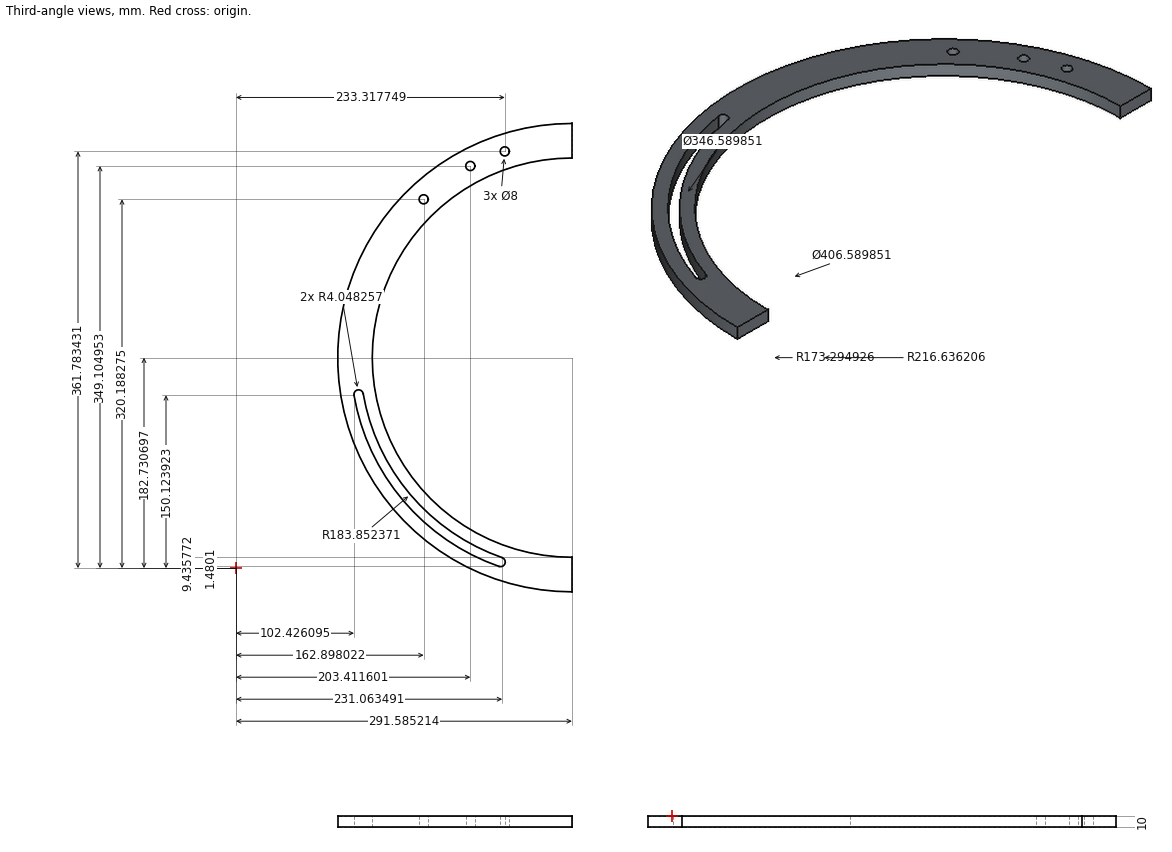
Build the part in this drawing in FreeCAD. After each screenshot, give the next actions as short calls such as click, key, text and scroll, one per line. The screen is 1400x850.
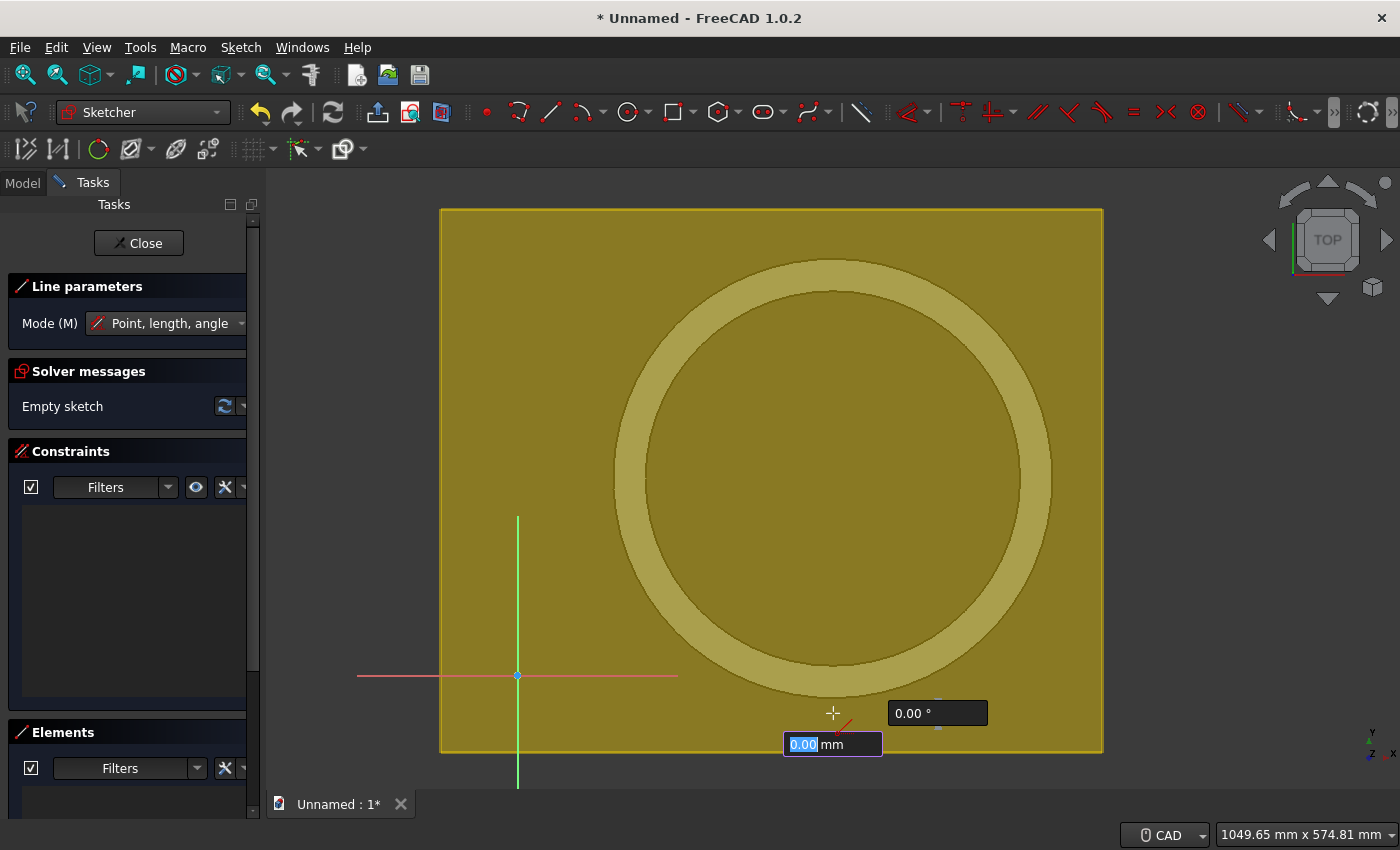
scroll(833, 666, up, 3)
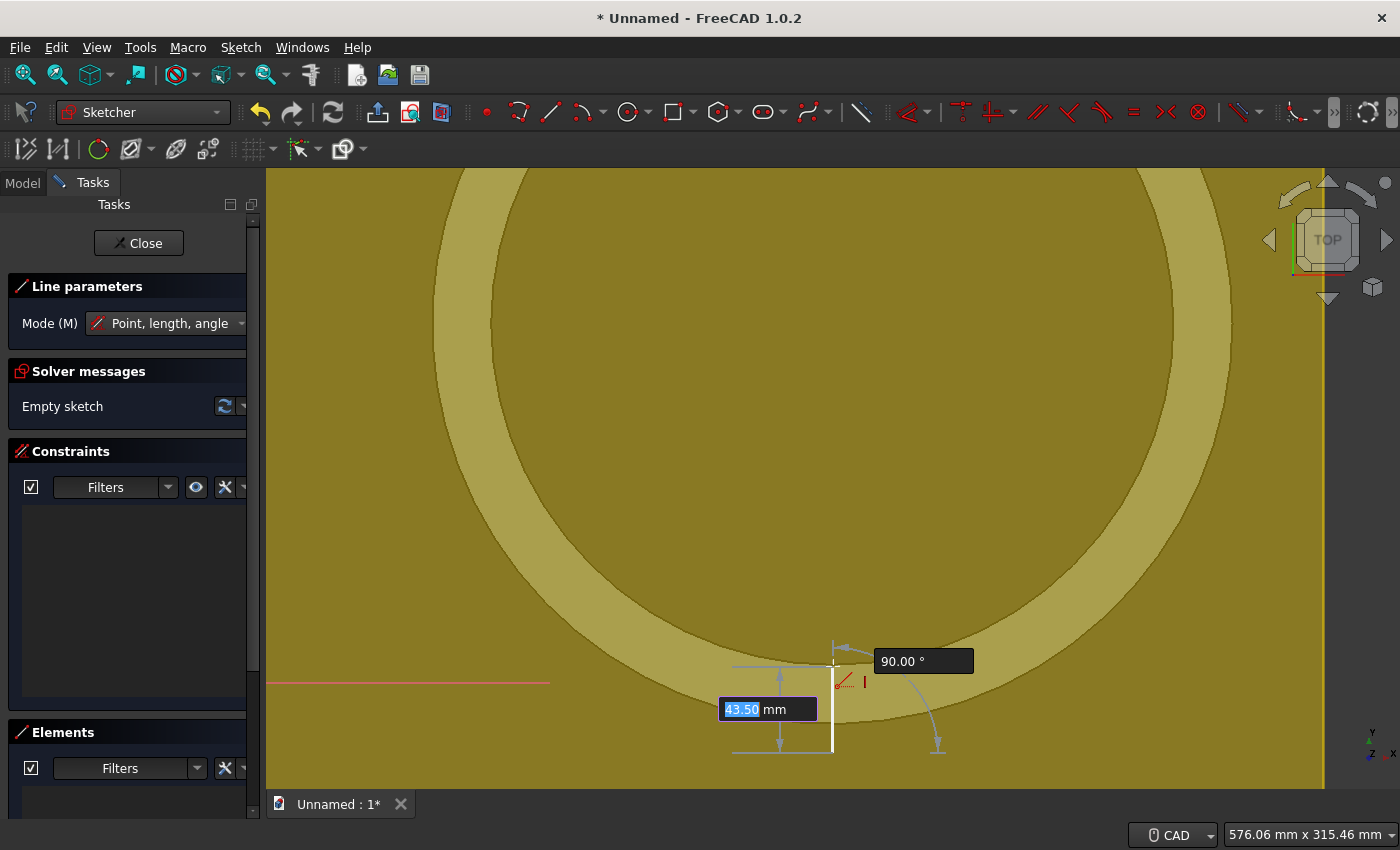
click(833, 665)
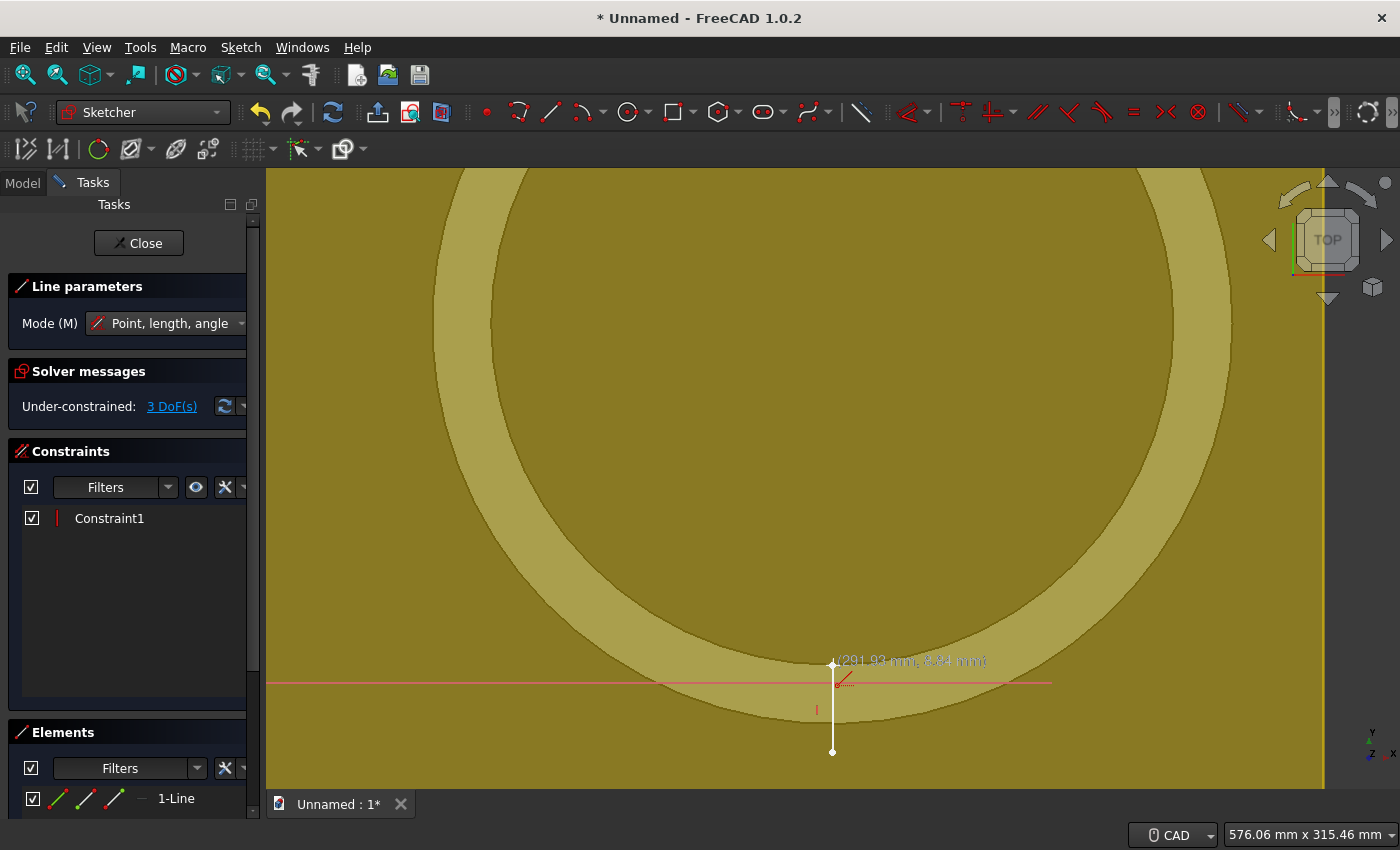
scroll(769, 605, down, 4)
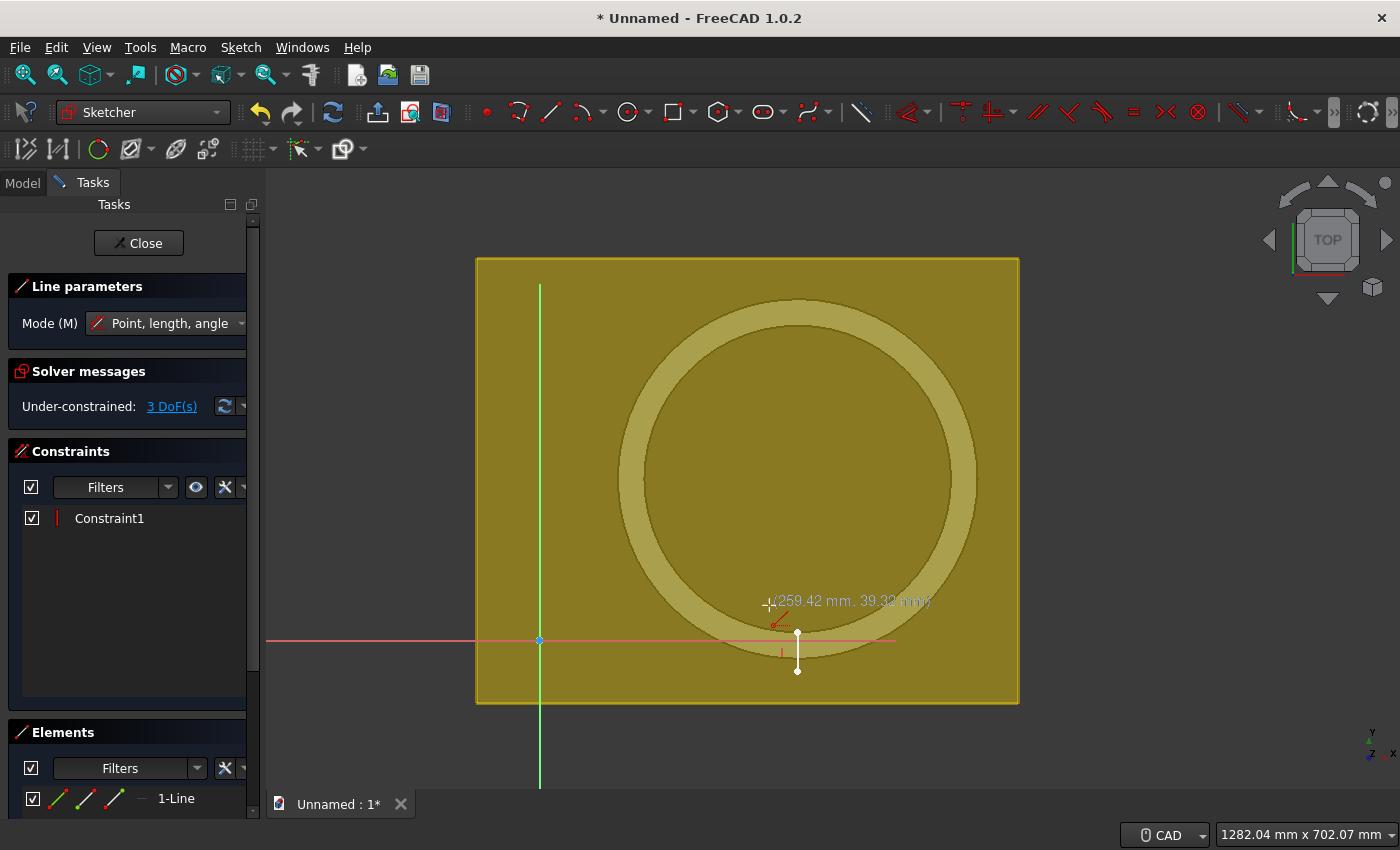
click(798, 326)
click(798, 287)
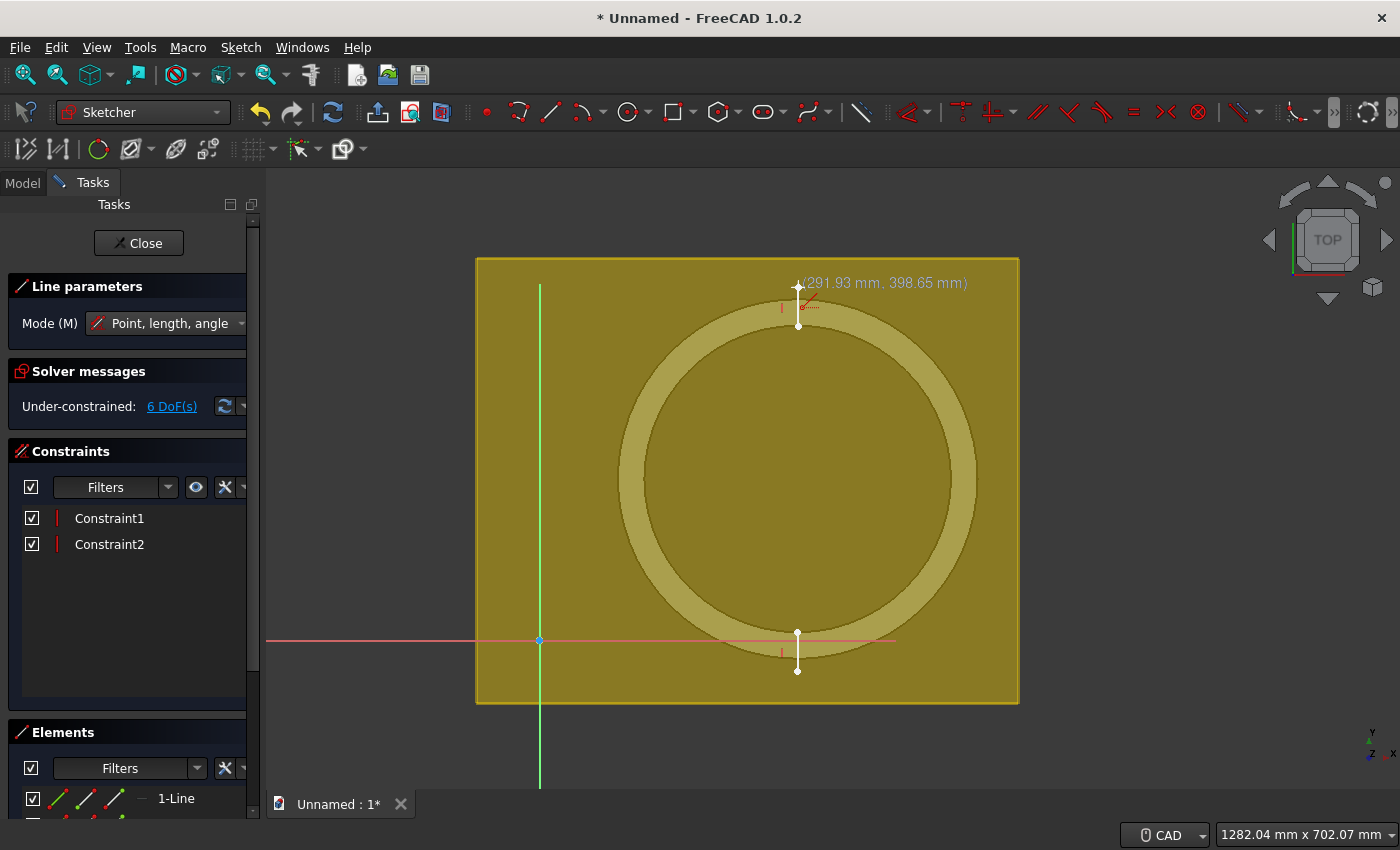
key(g)
key(3)
key(a)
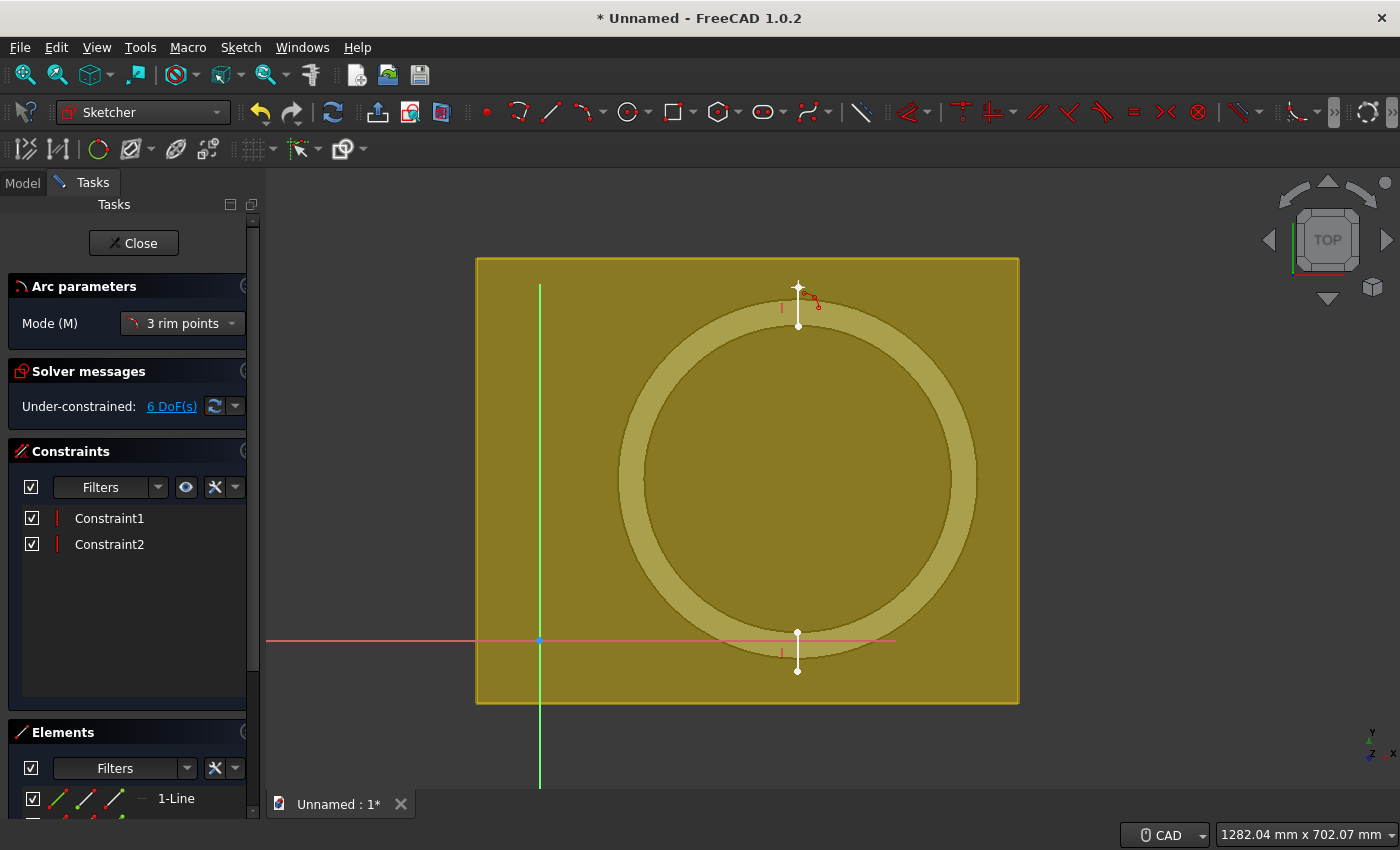
scroll(798, 632, up, 4)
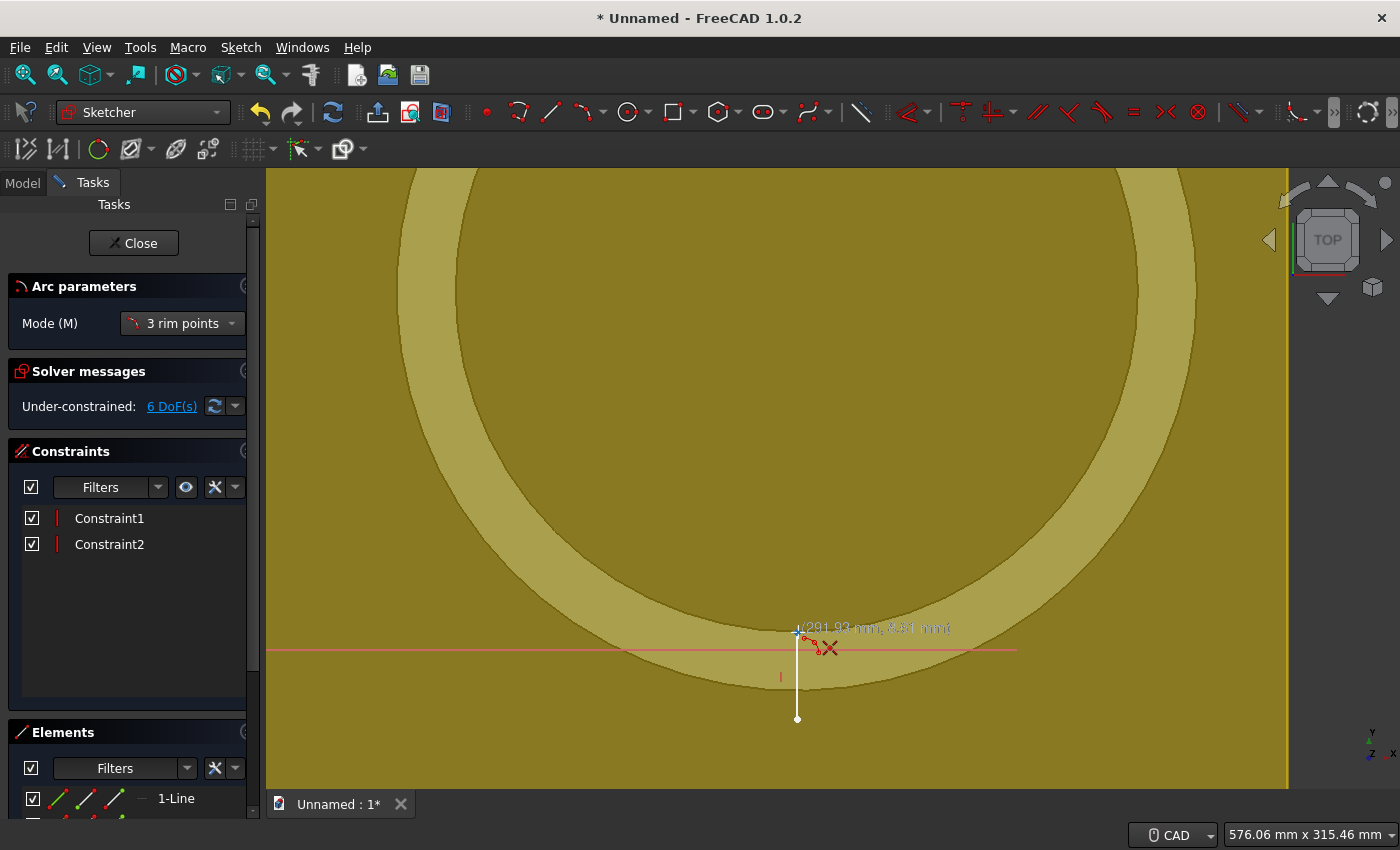
click(797, 633)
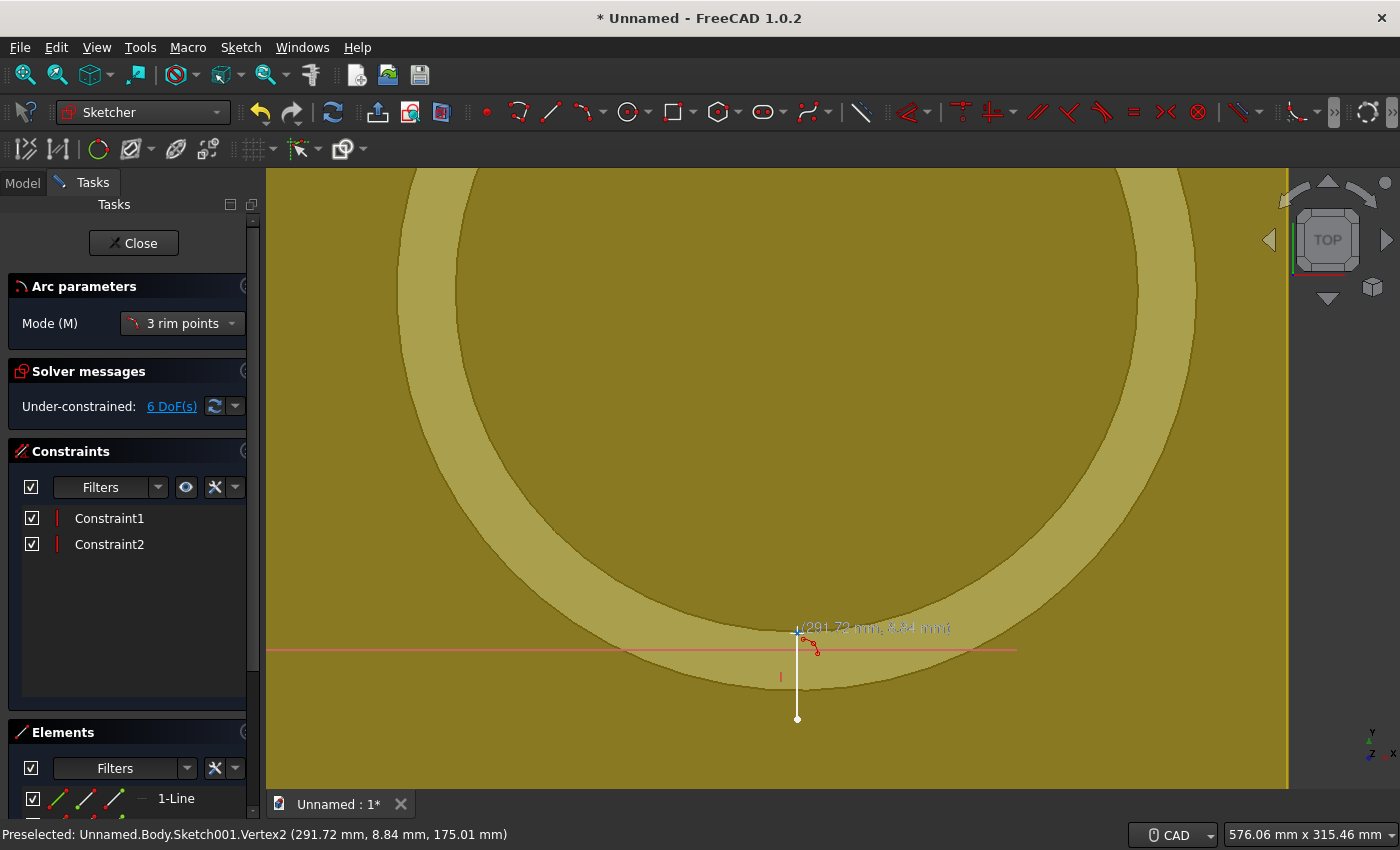
scroll(798, 632, down, 4)